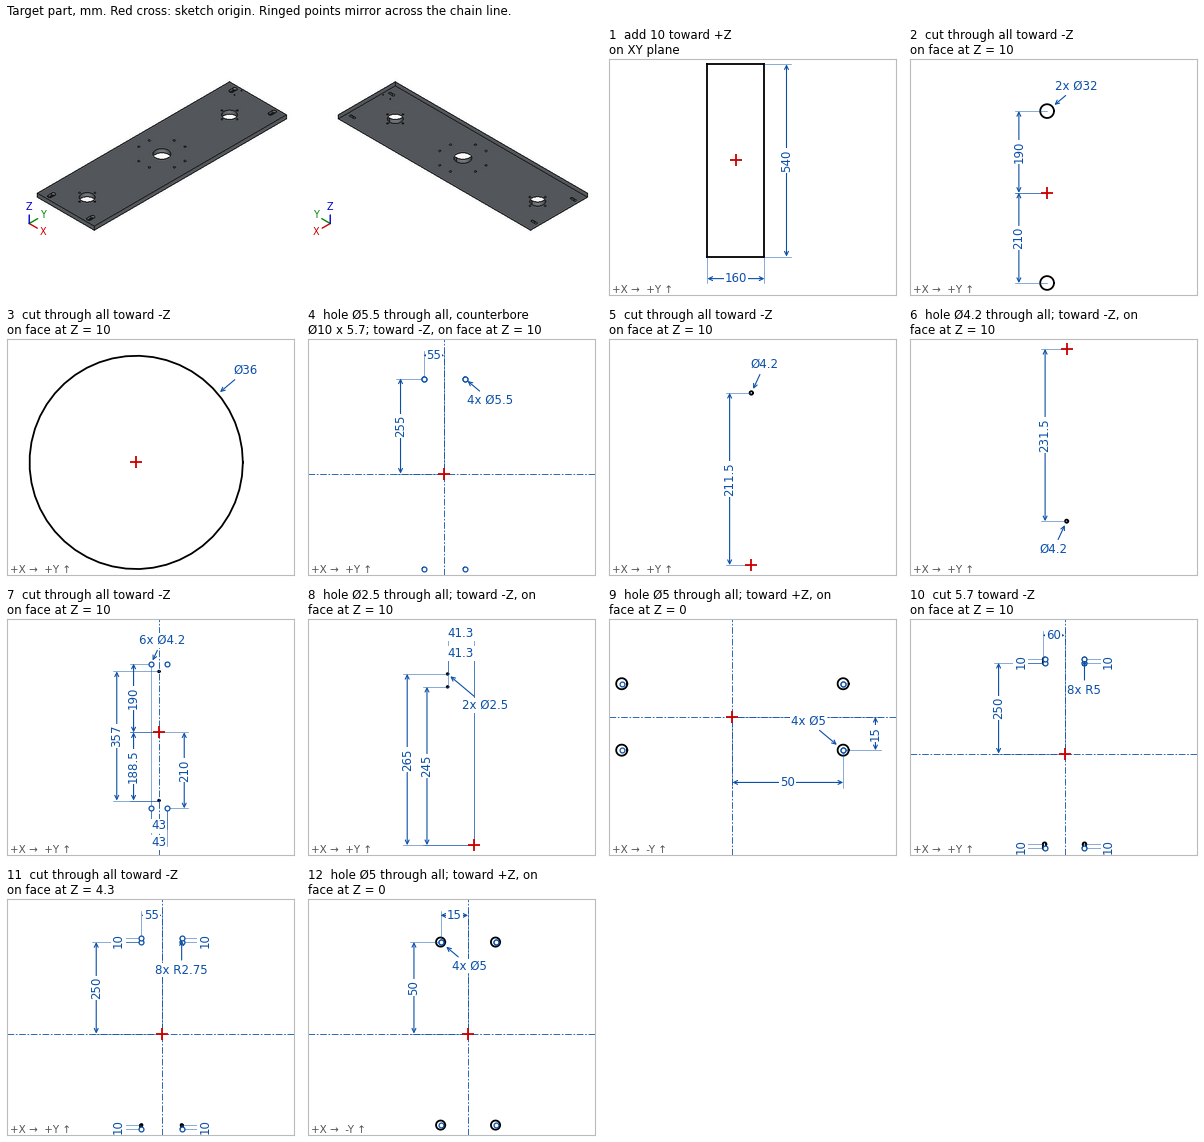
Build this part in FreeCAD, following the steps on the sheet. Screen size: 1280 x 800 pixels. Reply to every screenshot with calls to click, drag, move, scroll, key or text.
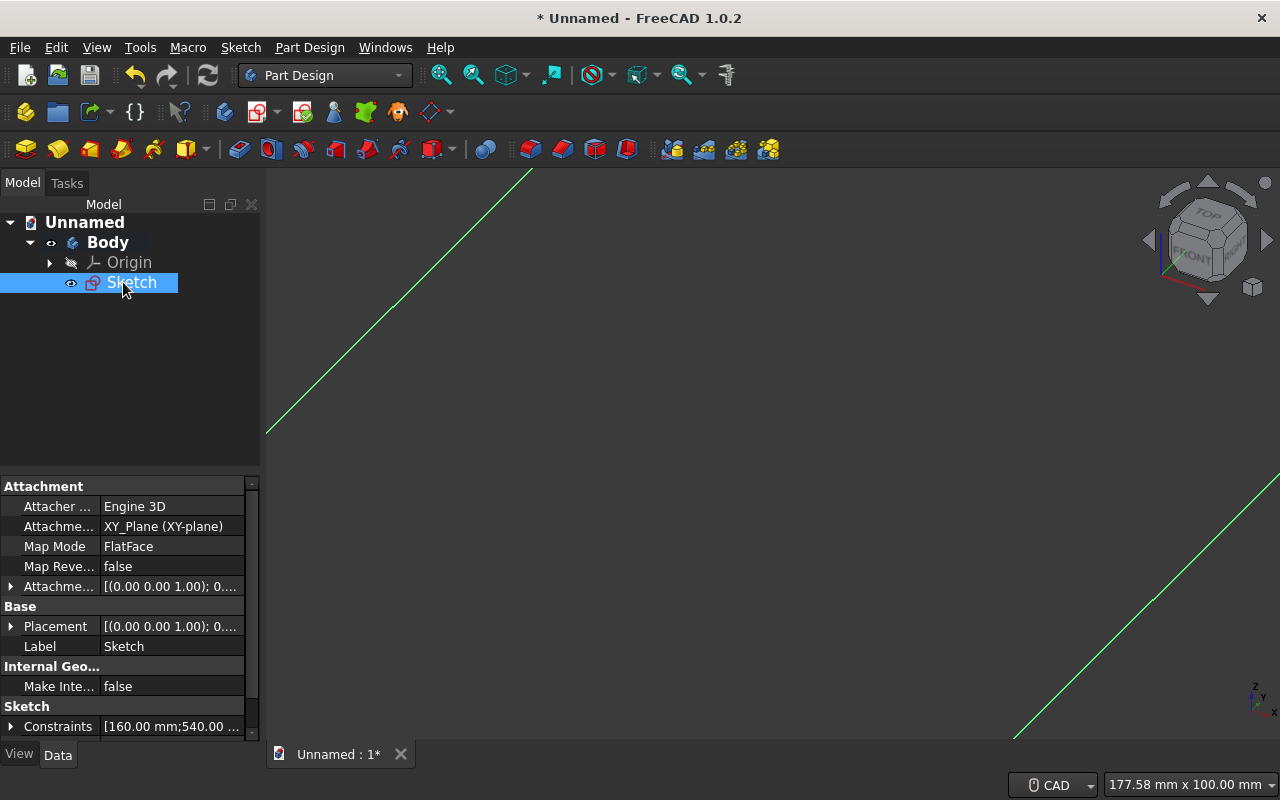
click(26, 150)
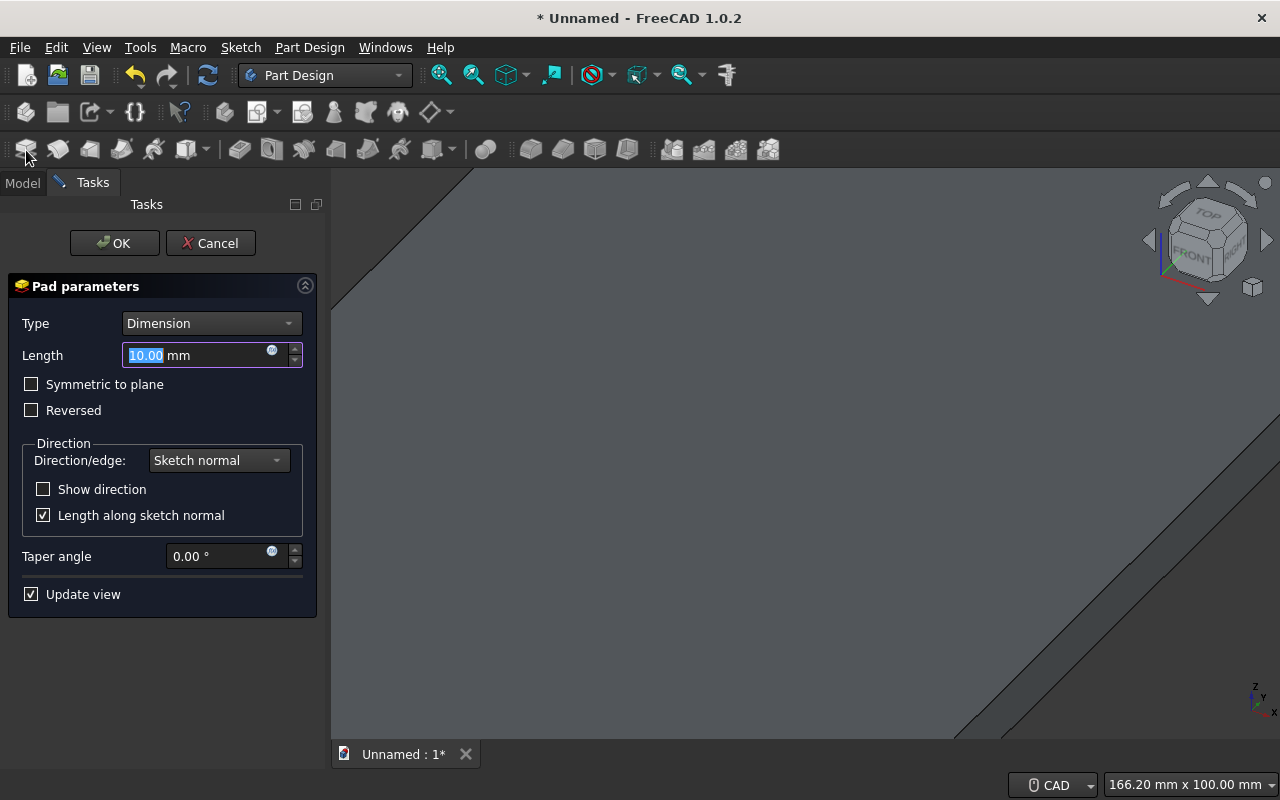
text(10)
key(Tab)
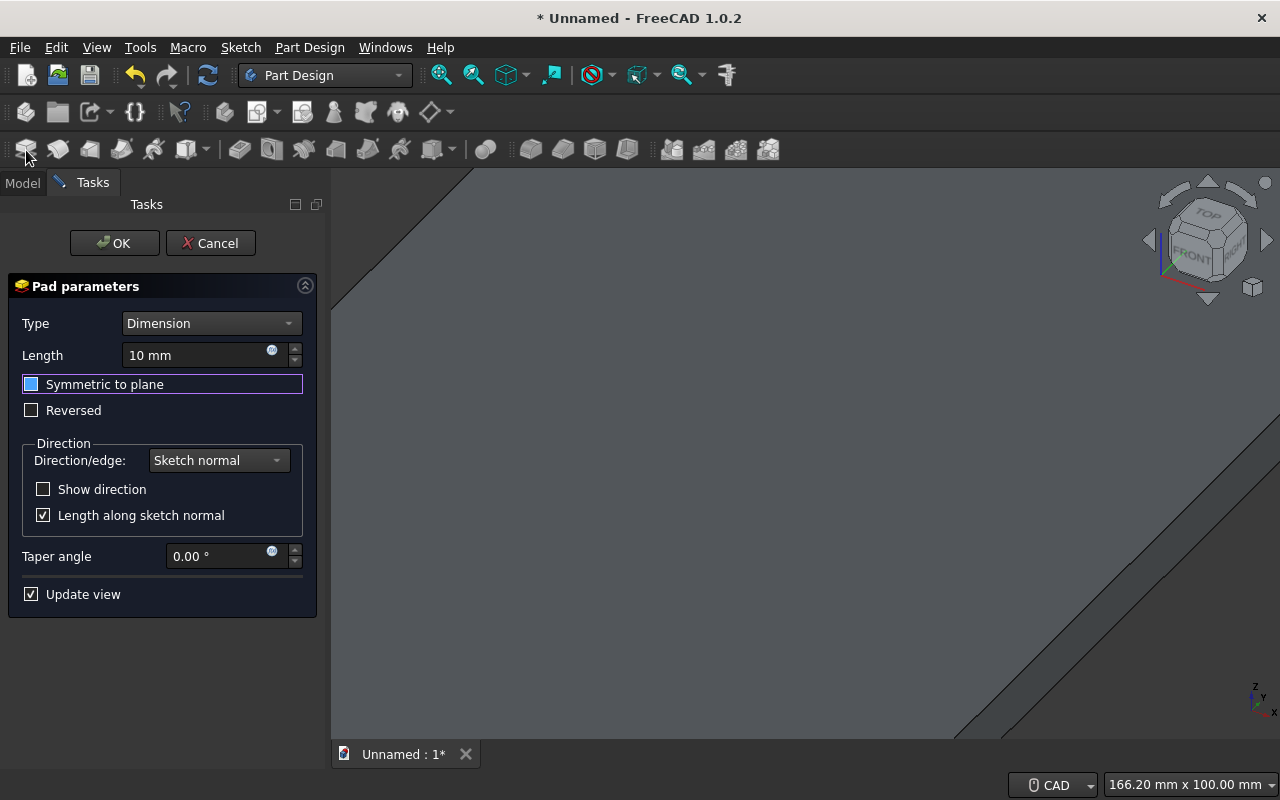
click(115, 243)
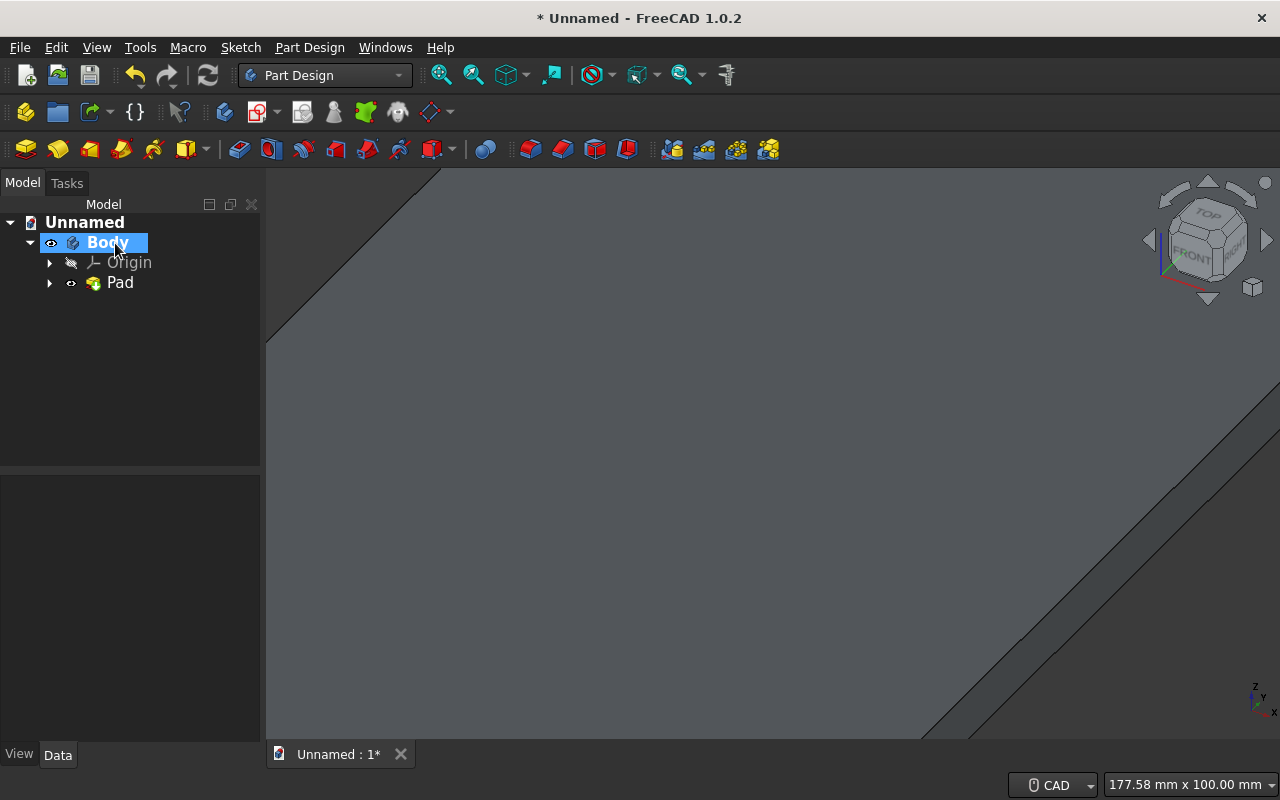
click(442, 76)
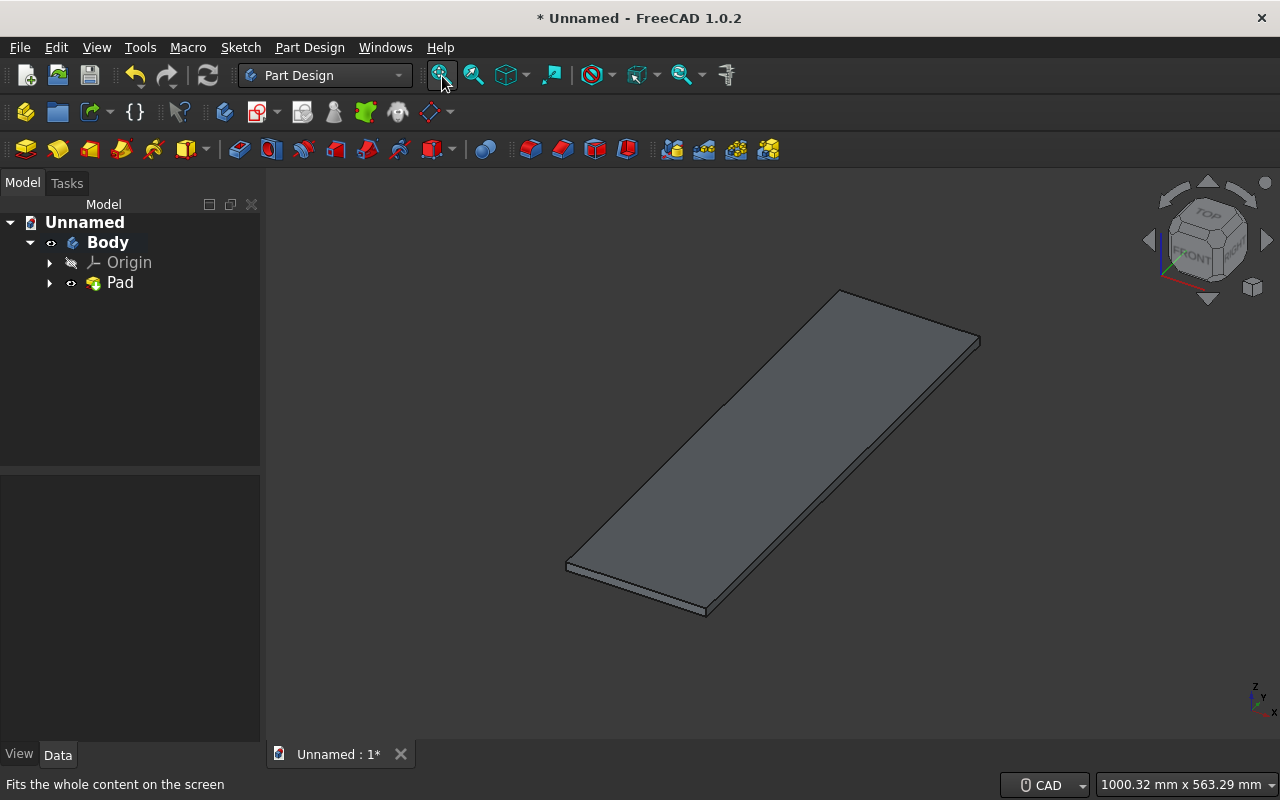
click(851, 371)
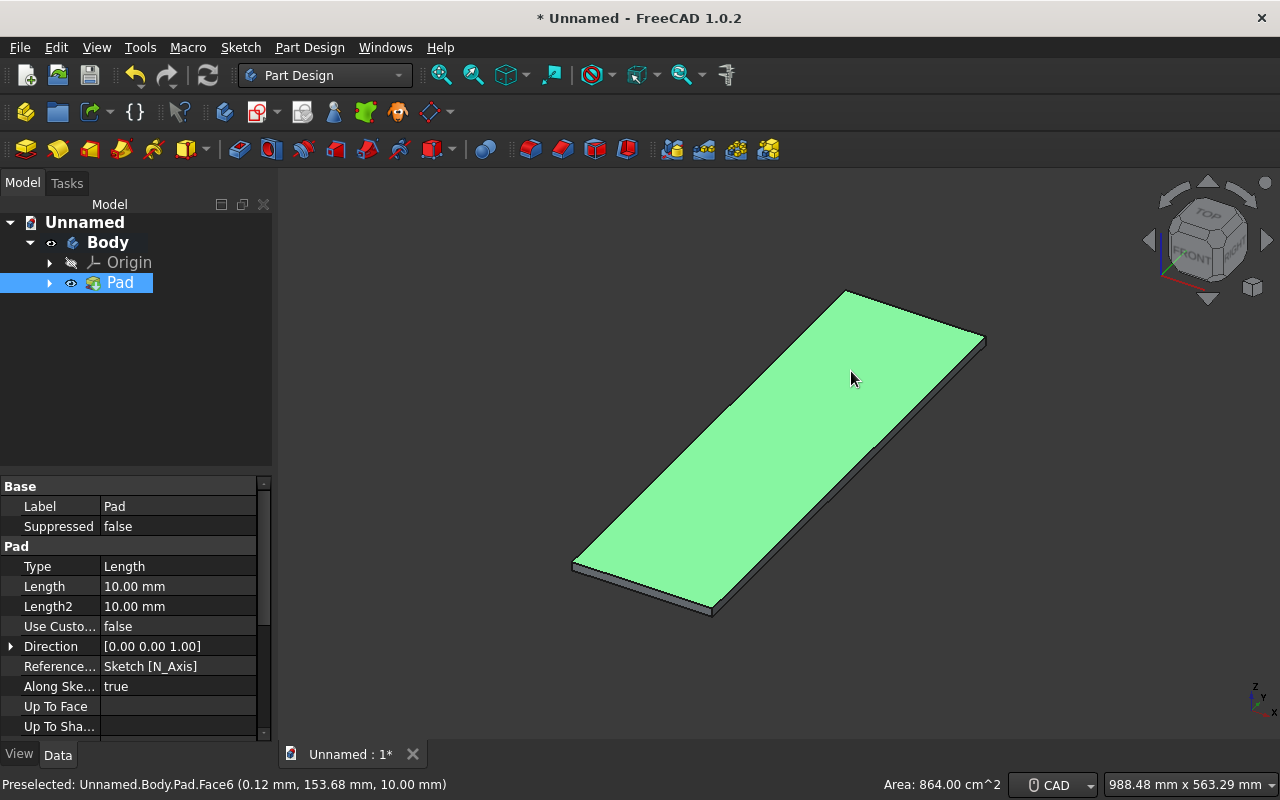
click(258, 112)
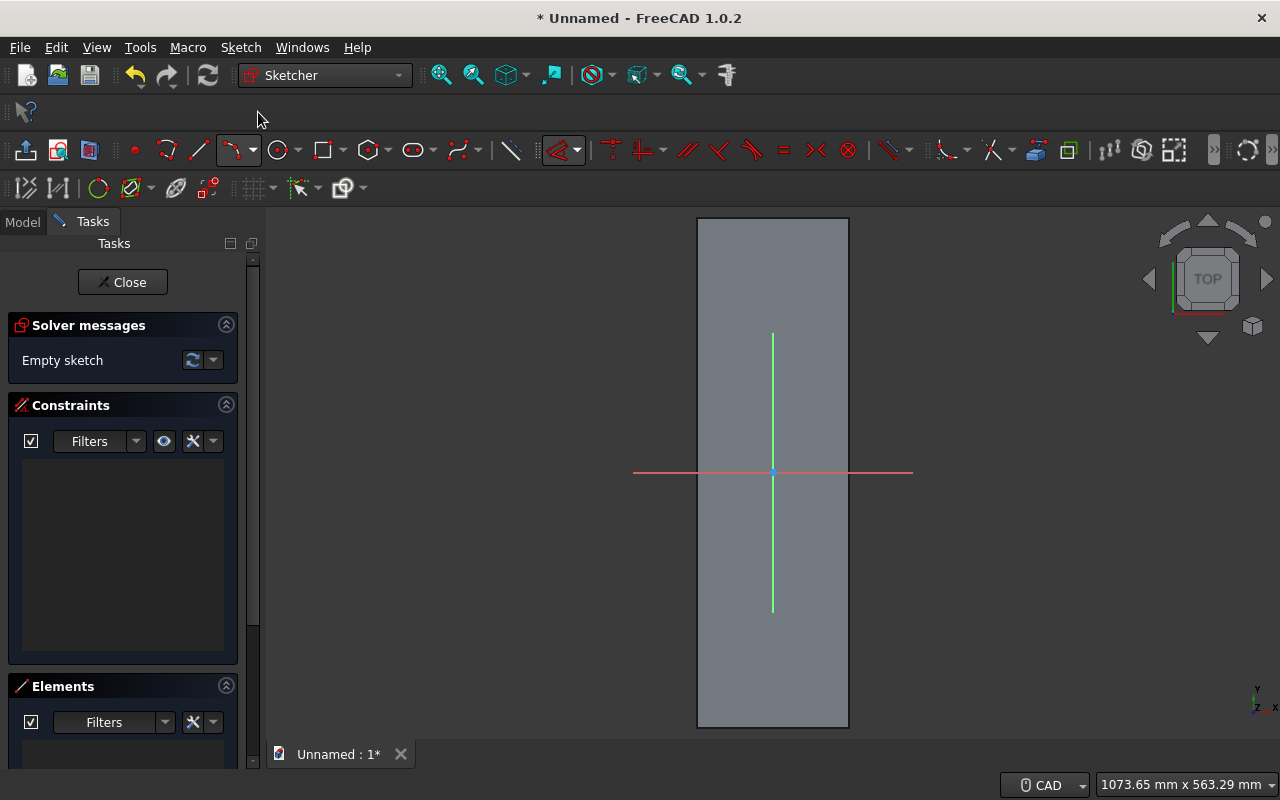
scroll(395, 430, down, 1)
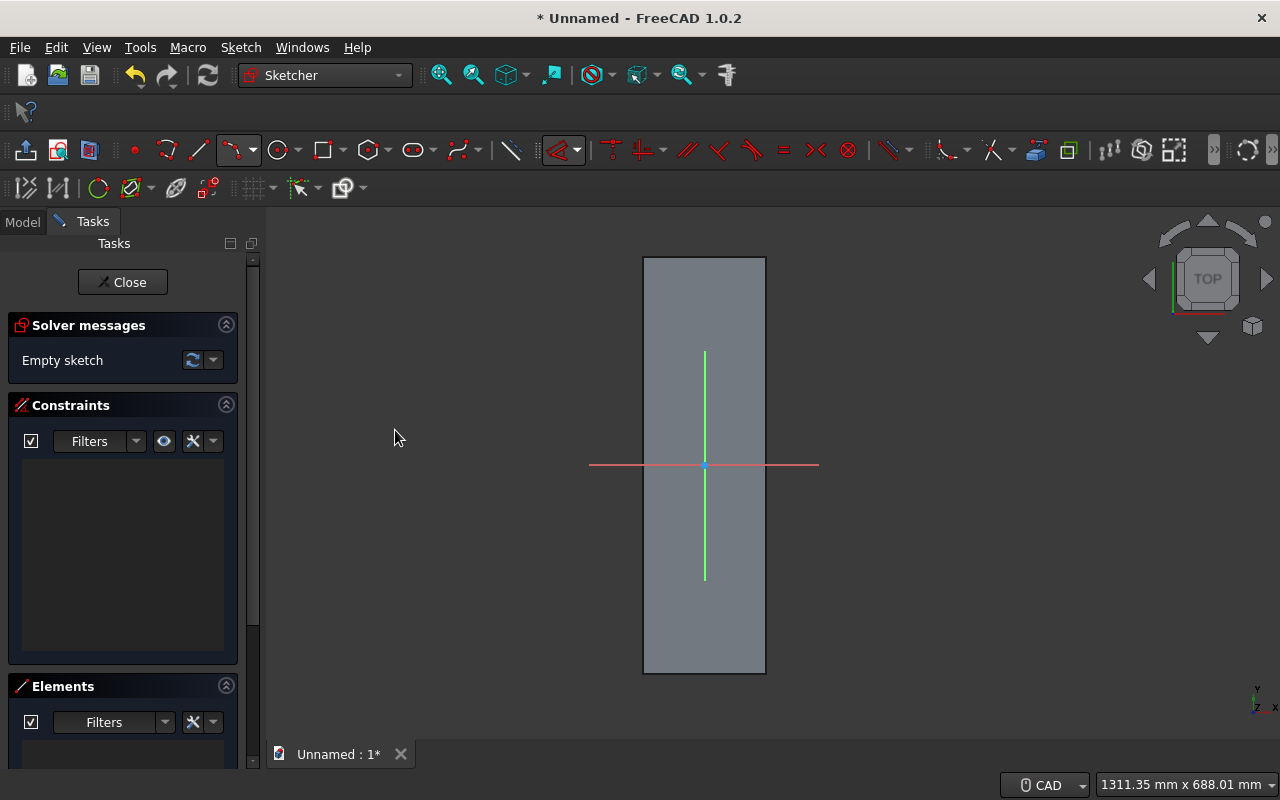
click(278, 150)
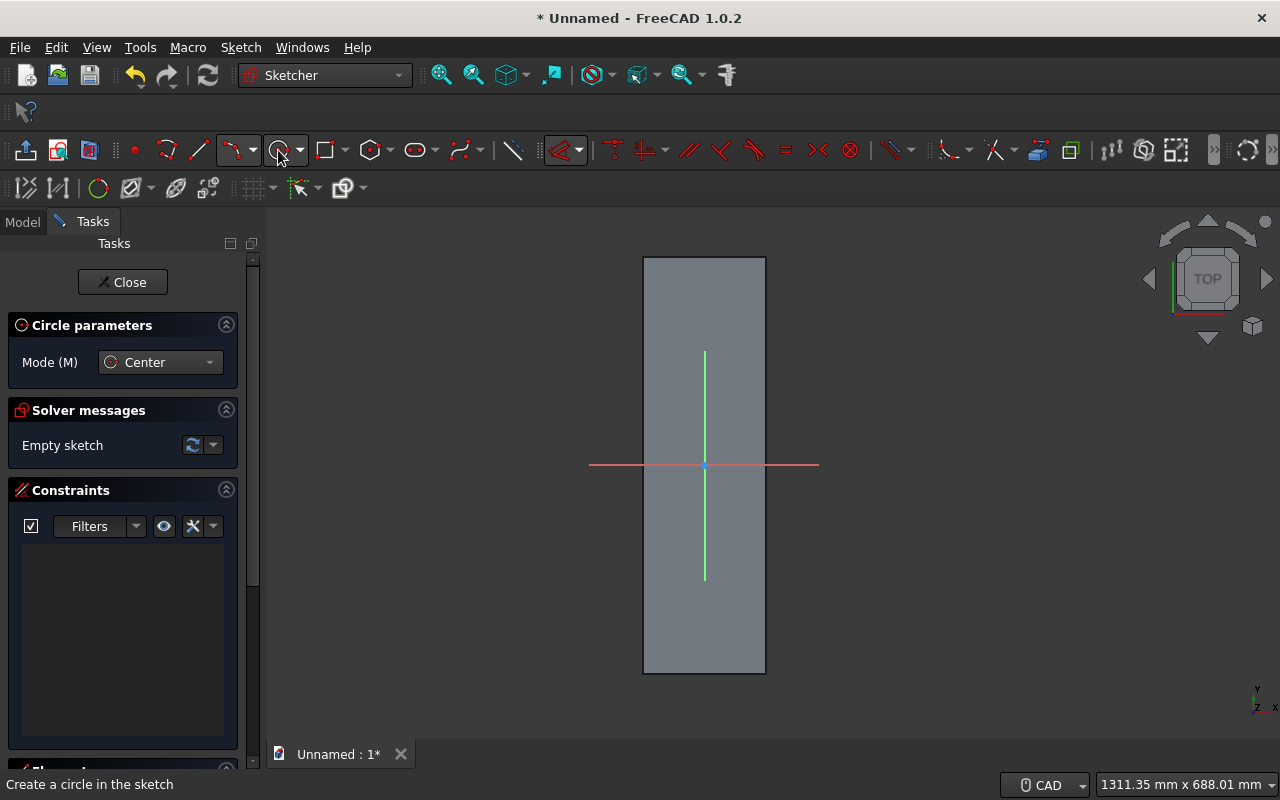
scroll(705, 318, up, 4)